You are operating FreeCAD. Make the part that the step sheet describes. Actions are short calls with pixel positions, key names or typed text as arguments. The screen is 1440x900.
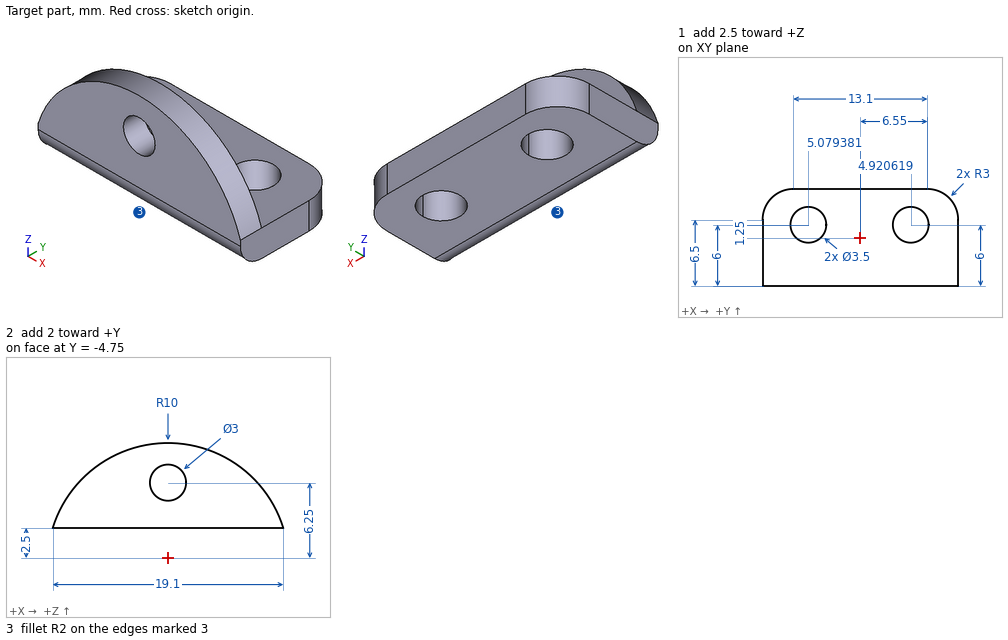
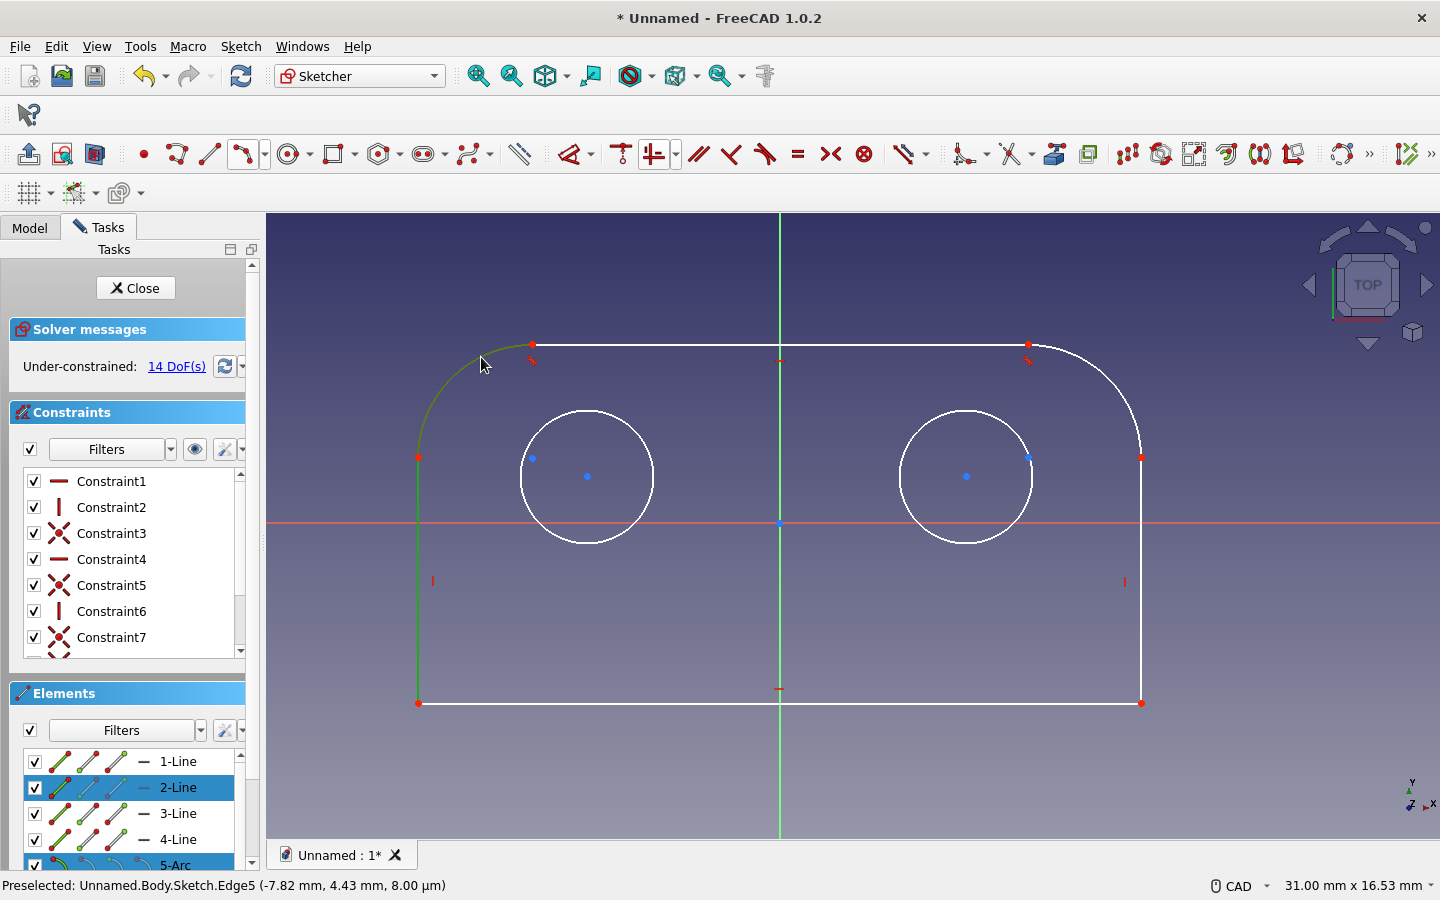
click(765, 154)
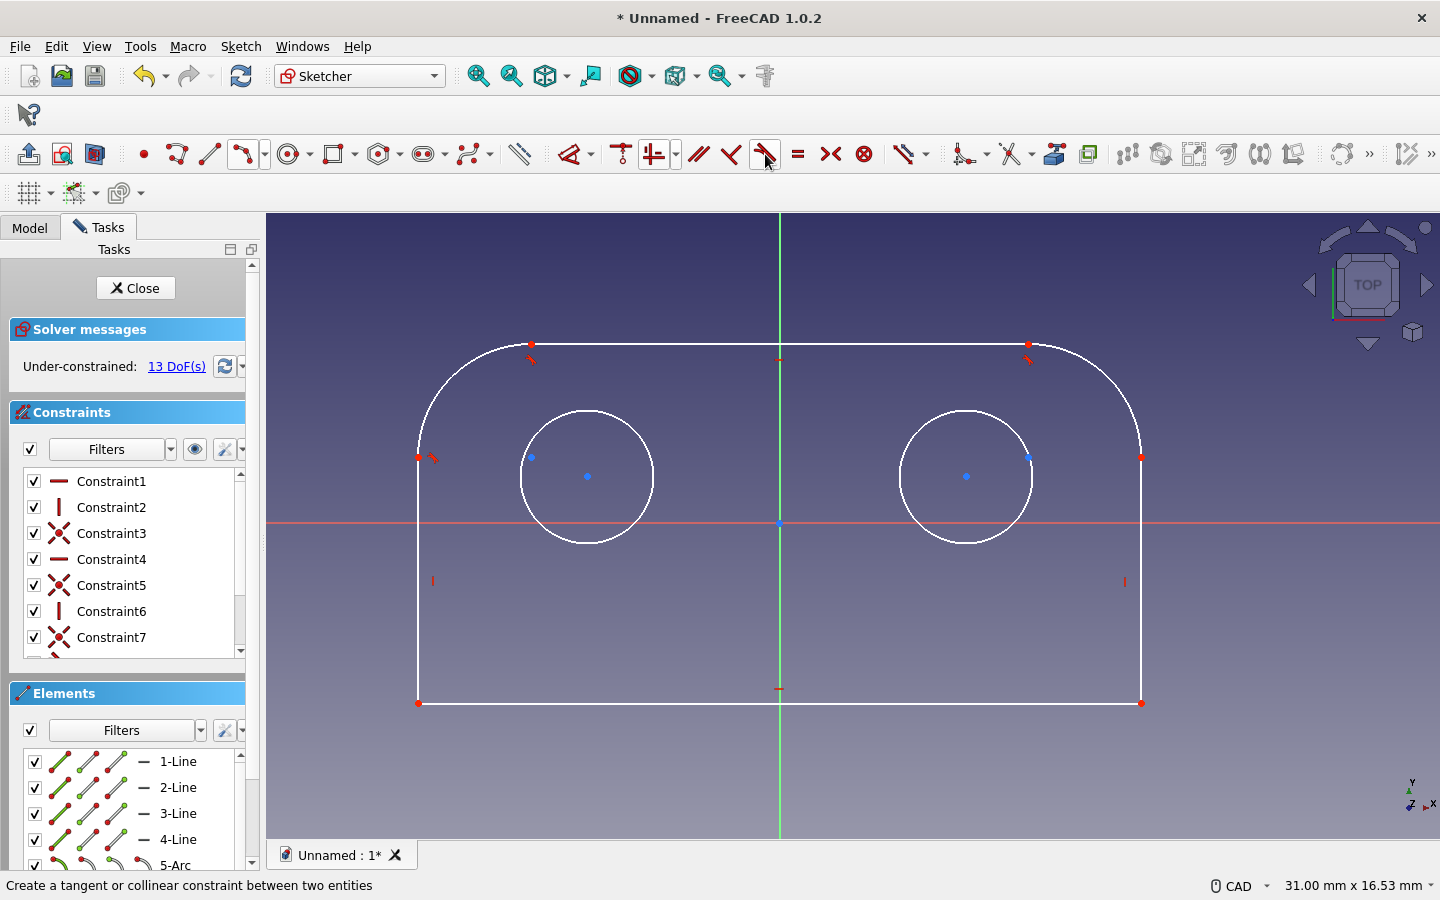
click(1141, 630)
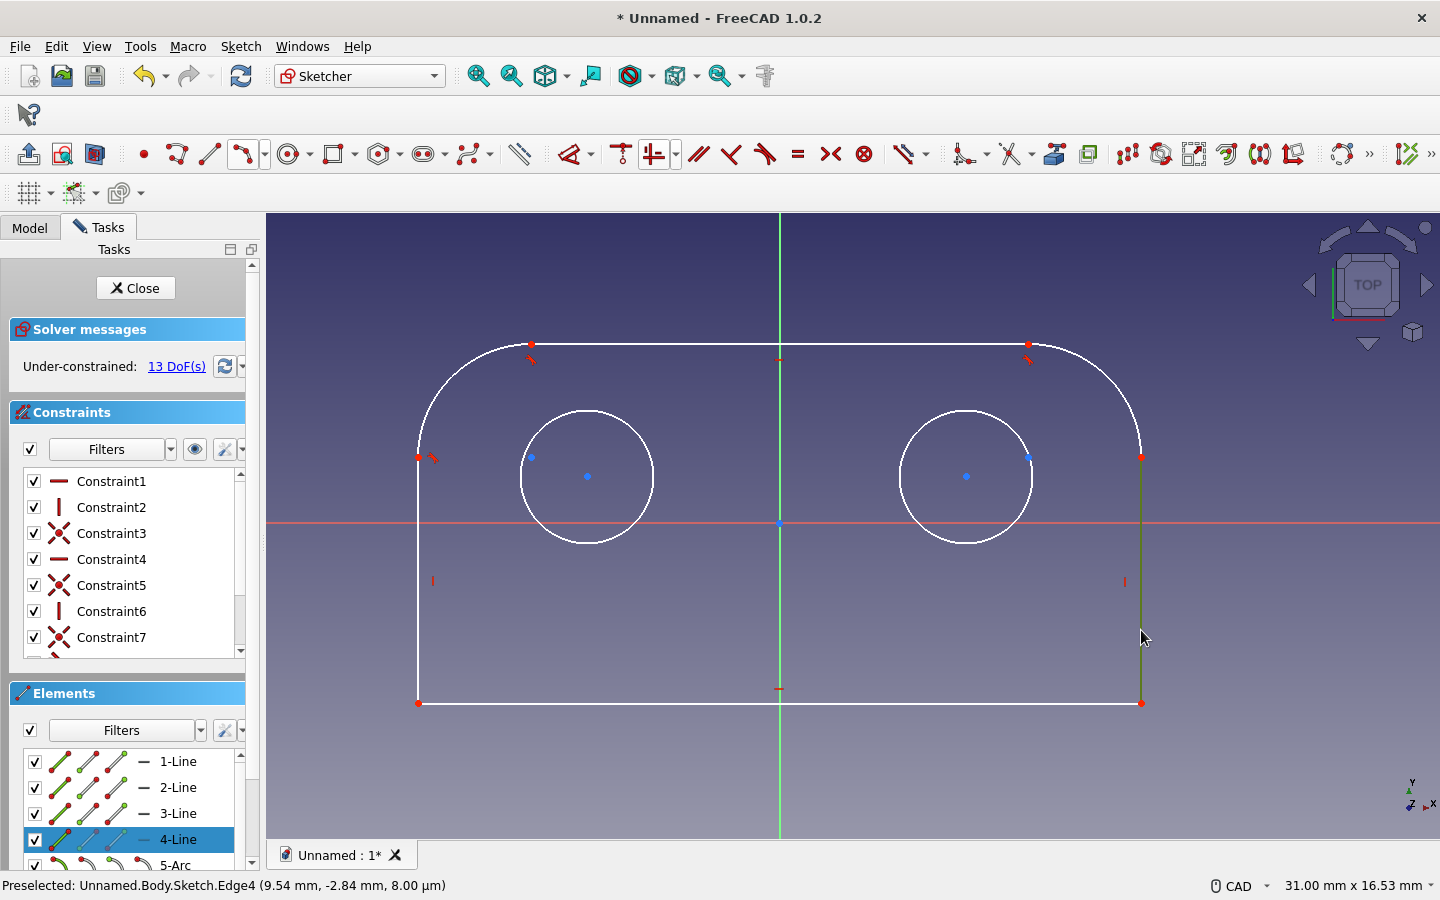
click(1129, 406)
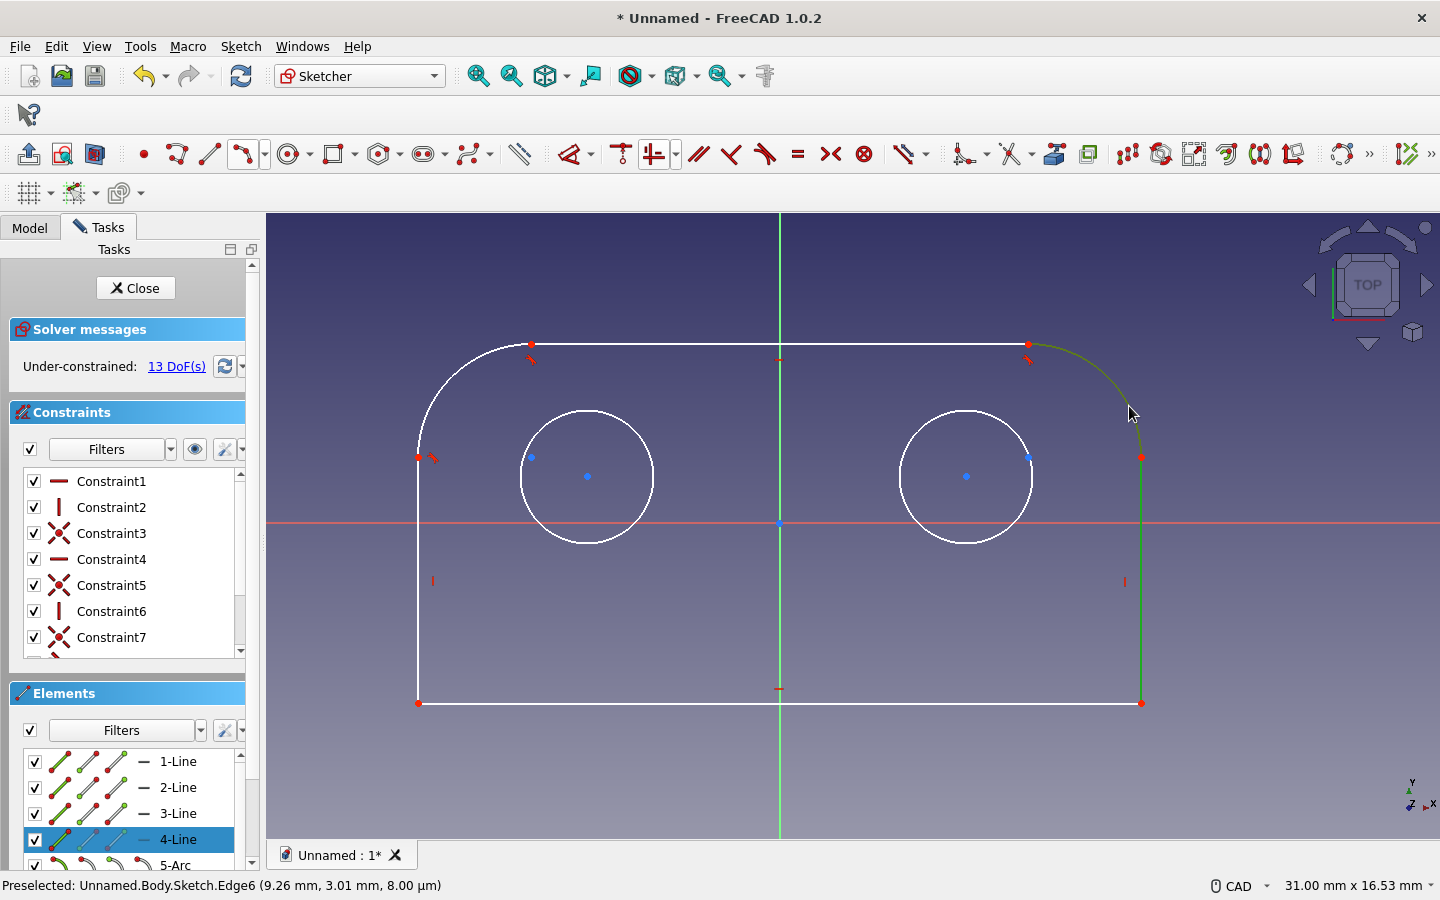
click(765, 154)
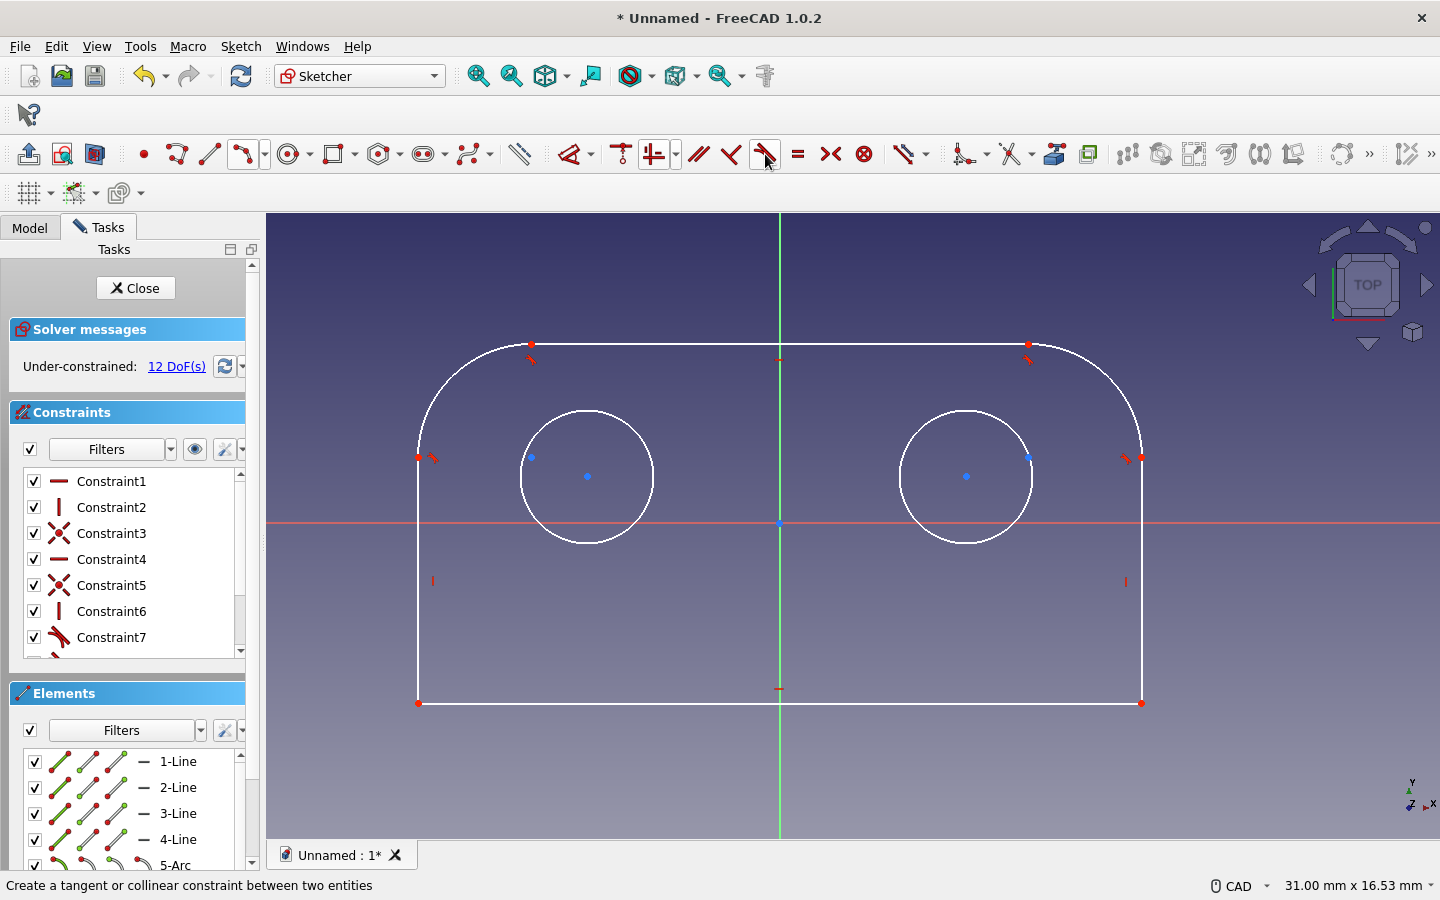
click(480, 356)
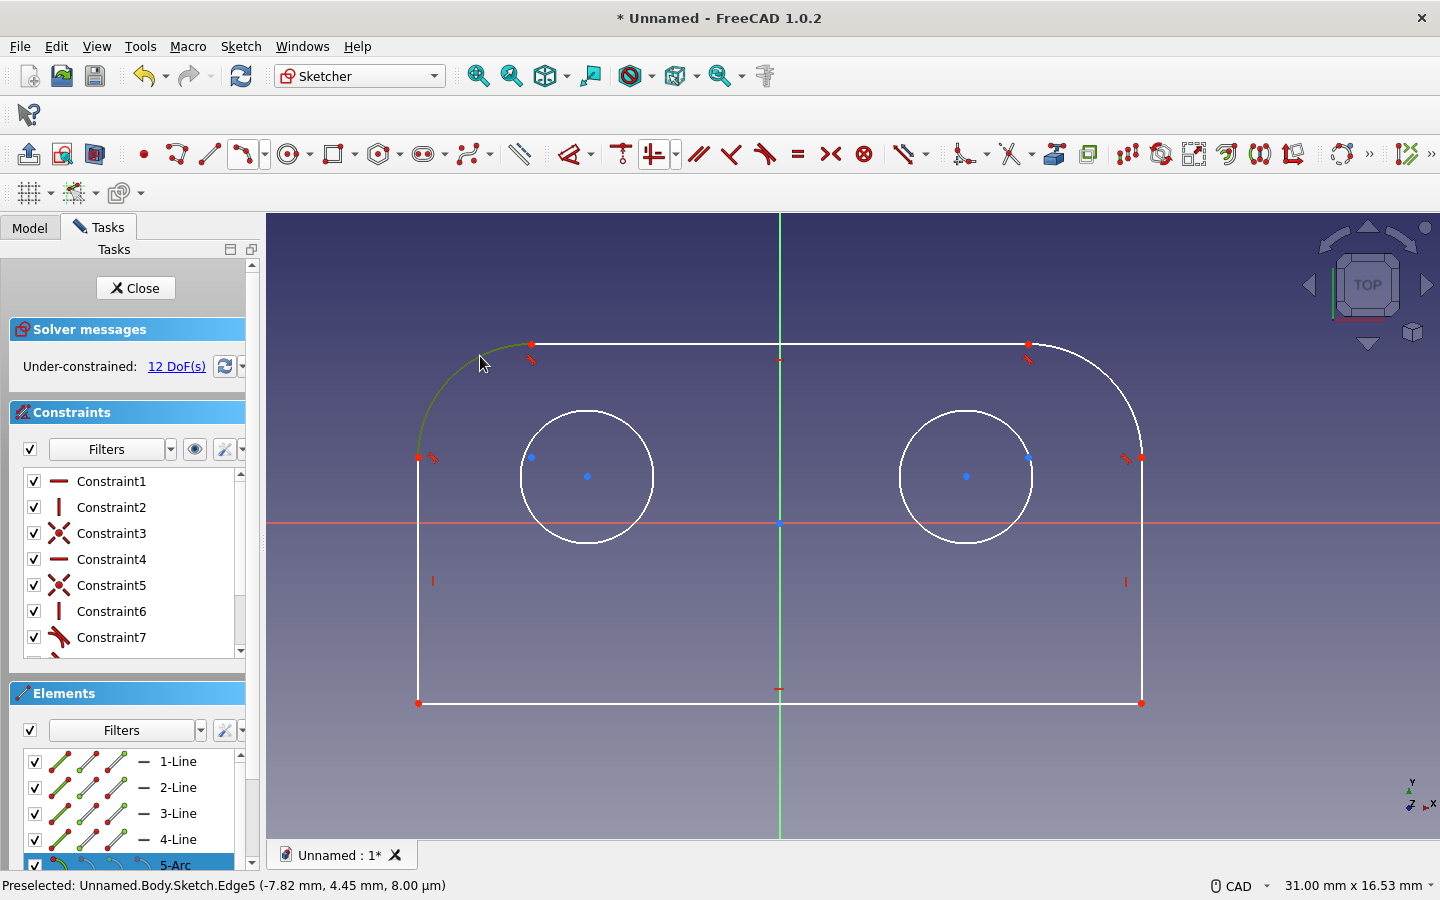
click(1130, 406)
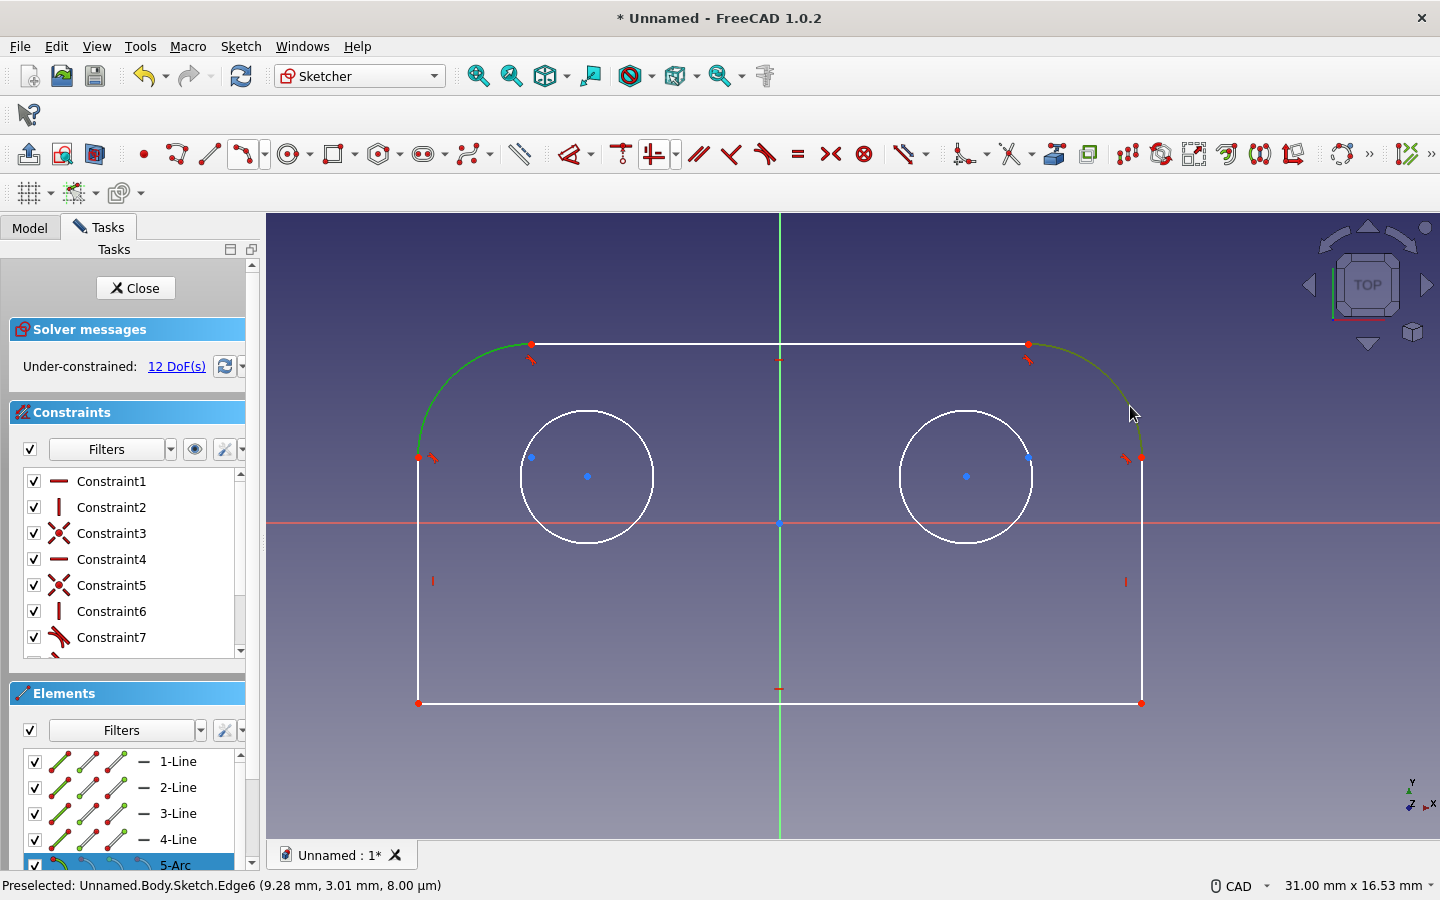
click(798, 154)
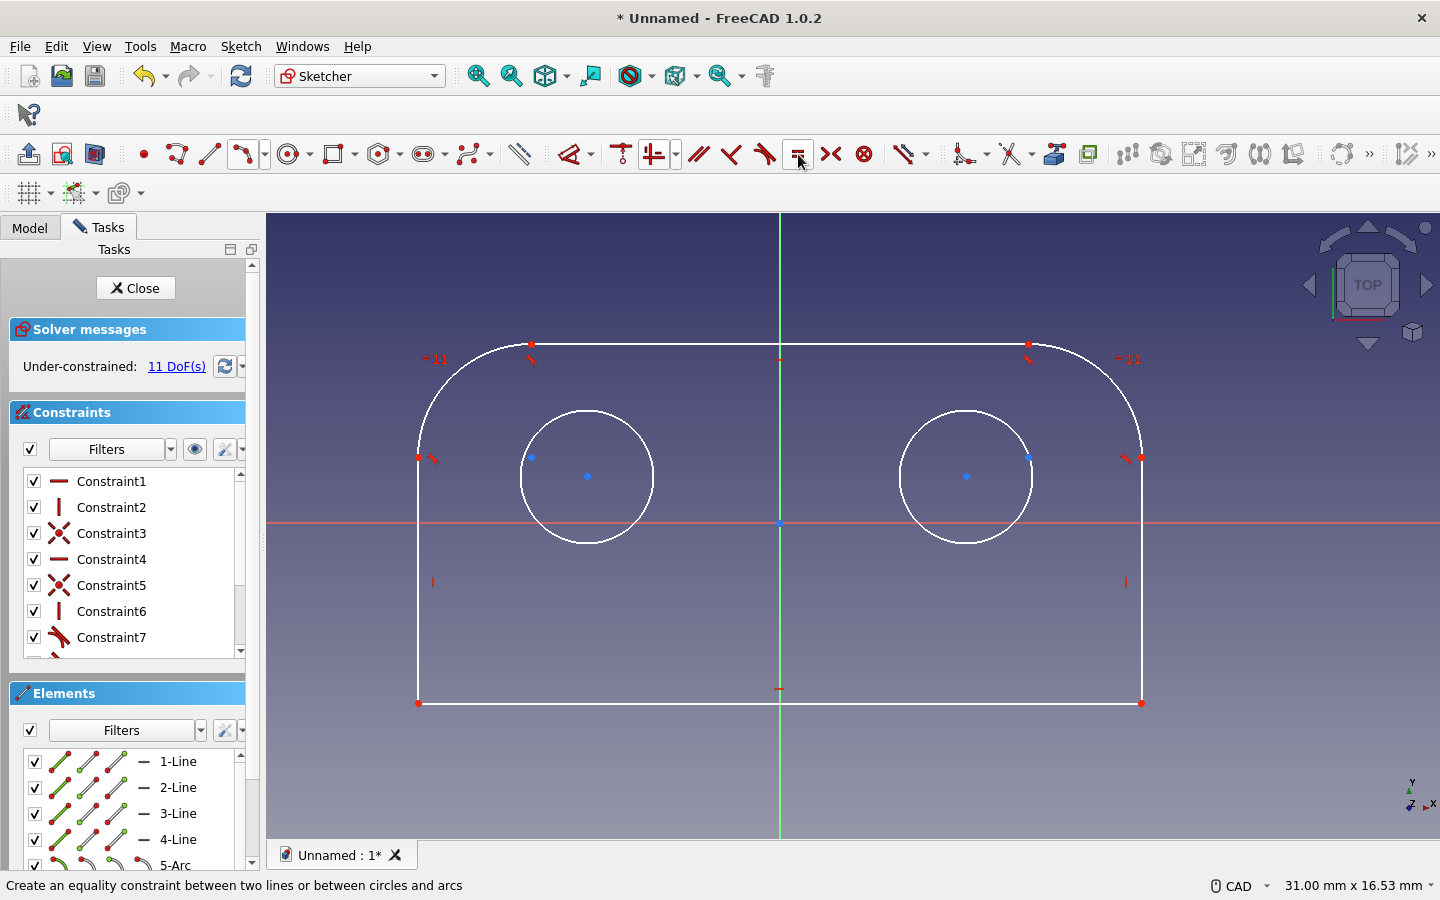
click(634, 430)